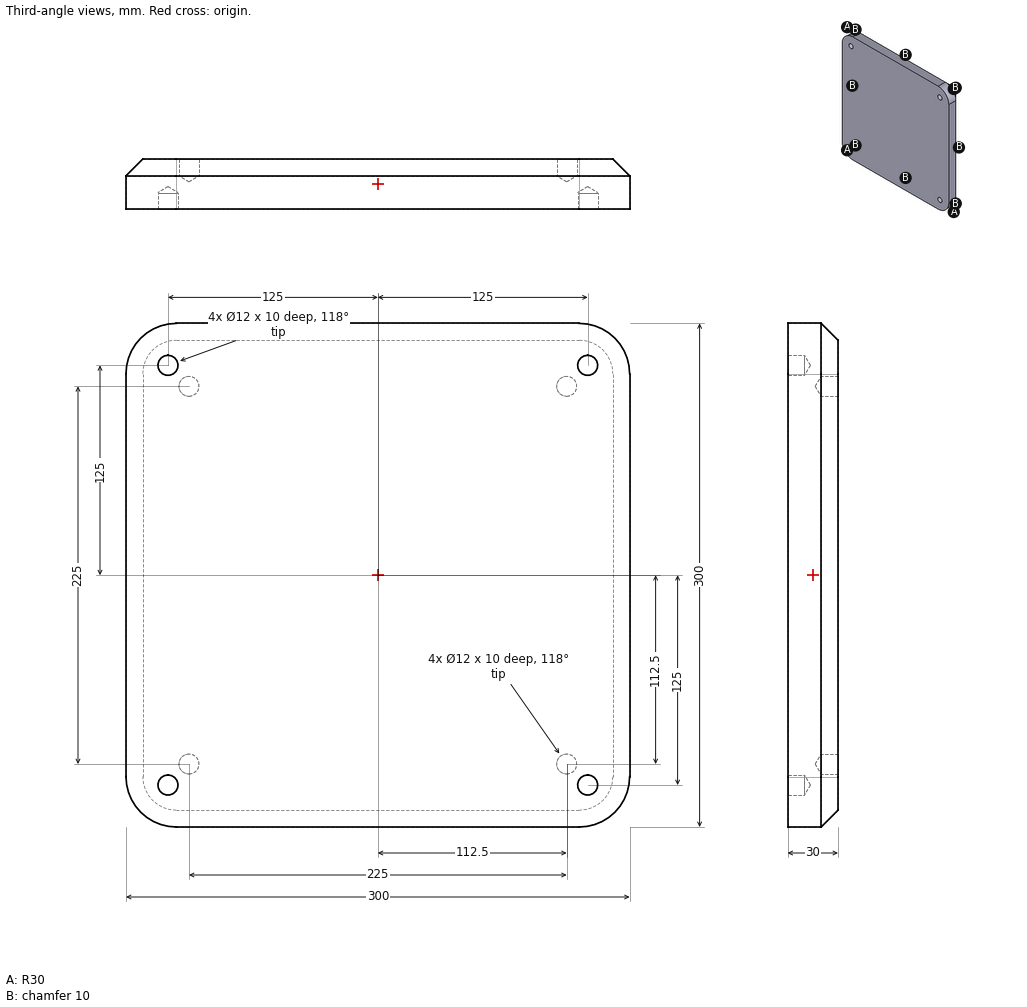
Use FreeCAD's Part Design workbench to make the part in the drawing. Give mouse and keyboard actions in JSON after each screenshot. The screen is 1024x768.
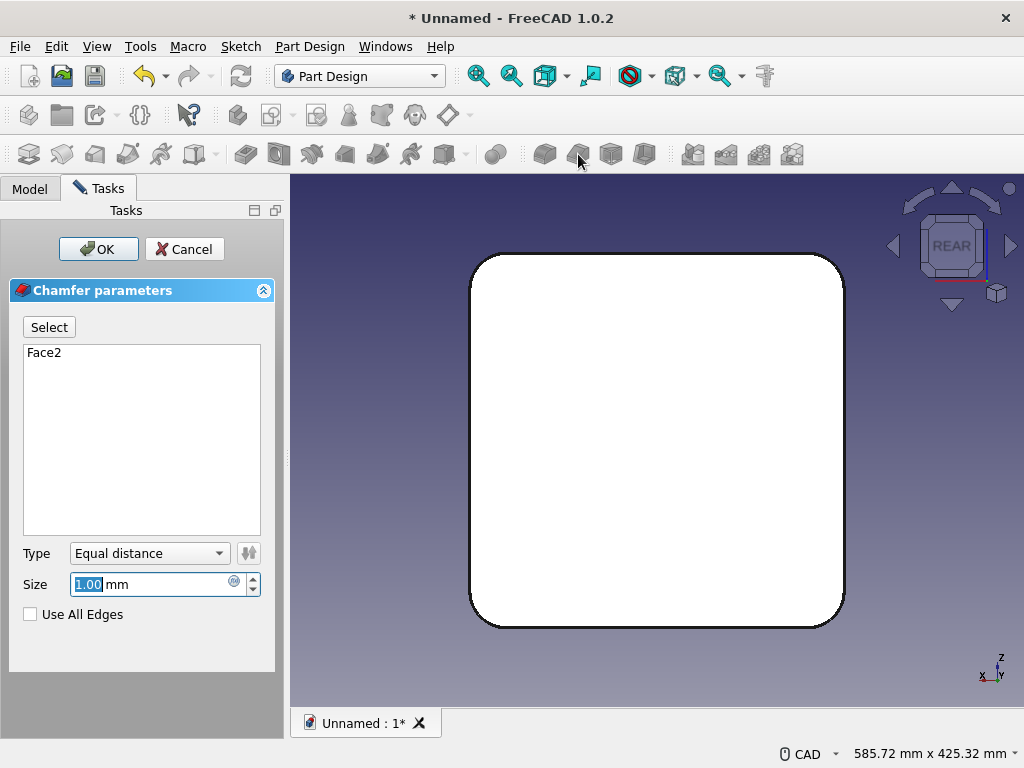
{"action": "type", "text": "10"}
{"action": "key", "text": "Tab"}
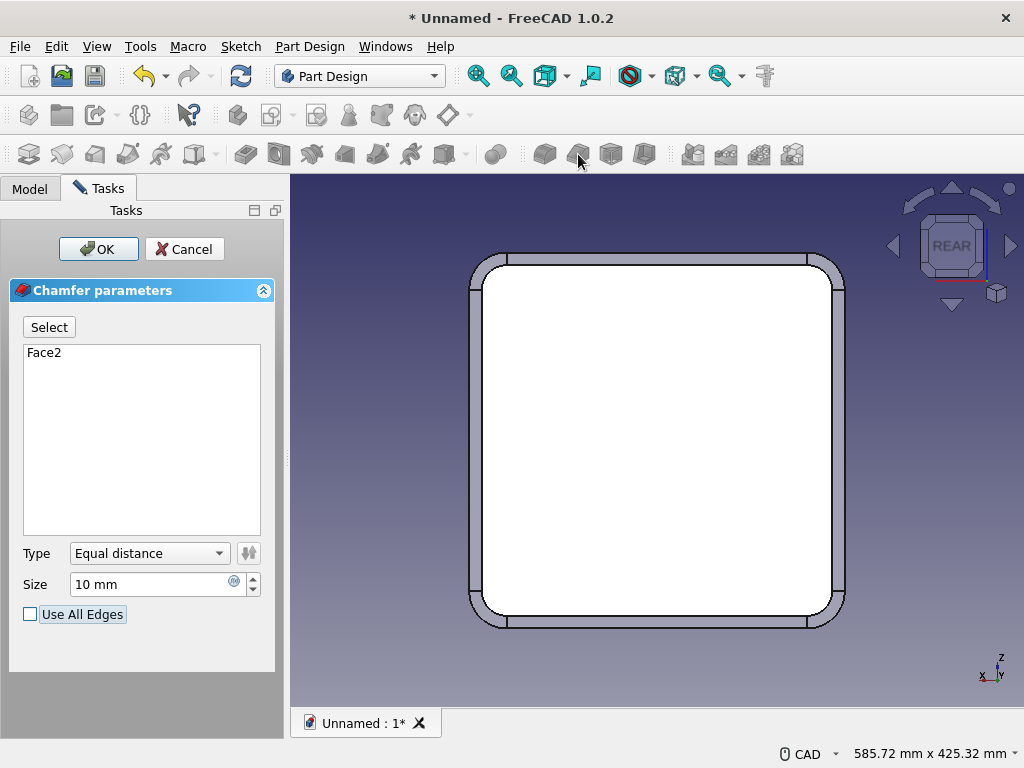
{"action": "left_click", "coordinate": [99, 249]}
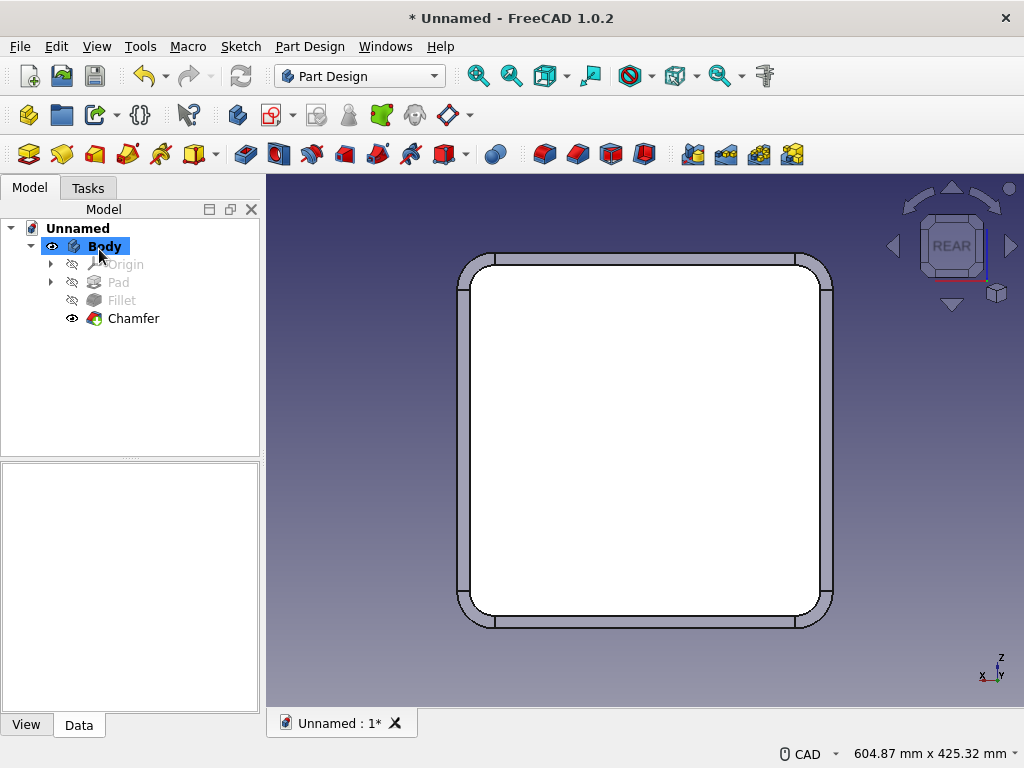
{"action": "left_click", "coordinate": [645, 439]}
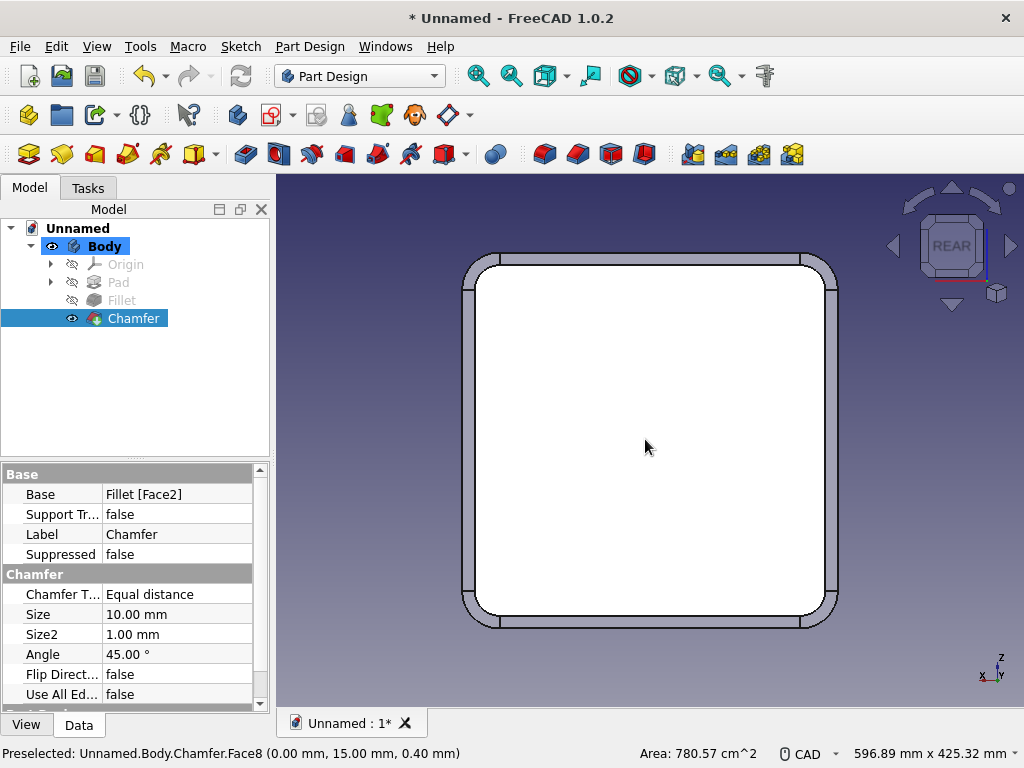
{"action": "left_click", "coordinate": [270, 116]}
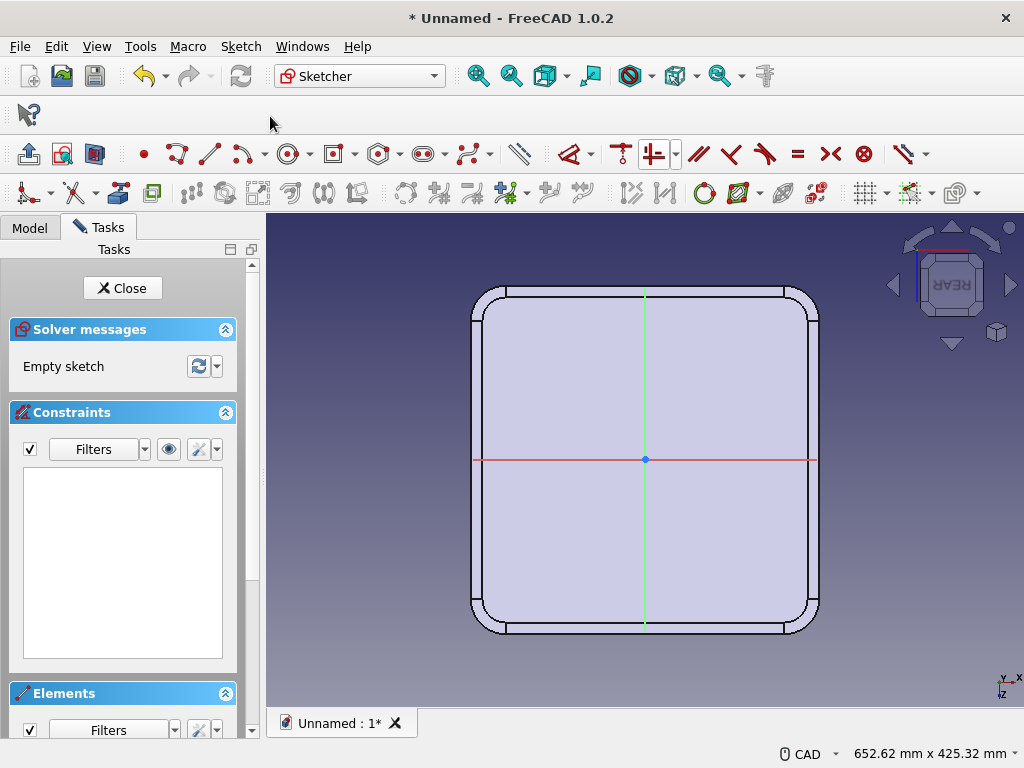
{"action": "left_click", "coordinate": [288, 154]}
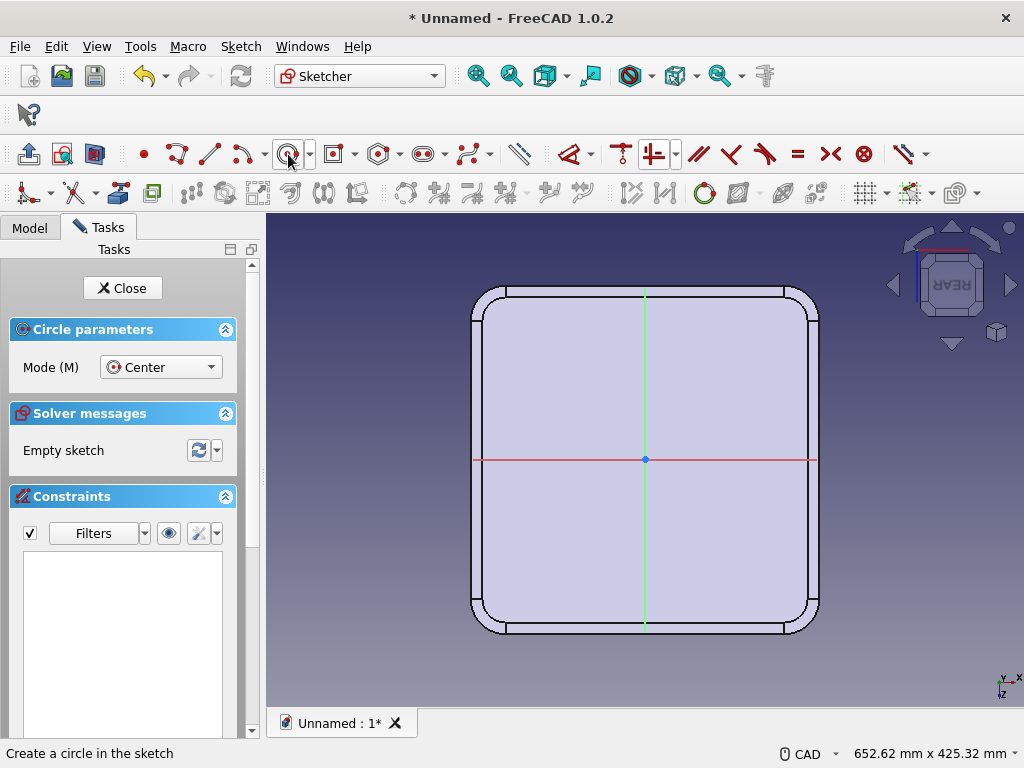
{"action": "scroll", "coordinate": [776, 329], "scroll_direction": "up", "scroll_amount": 6}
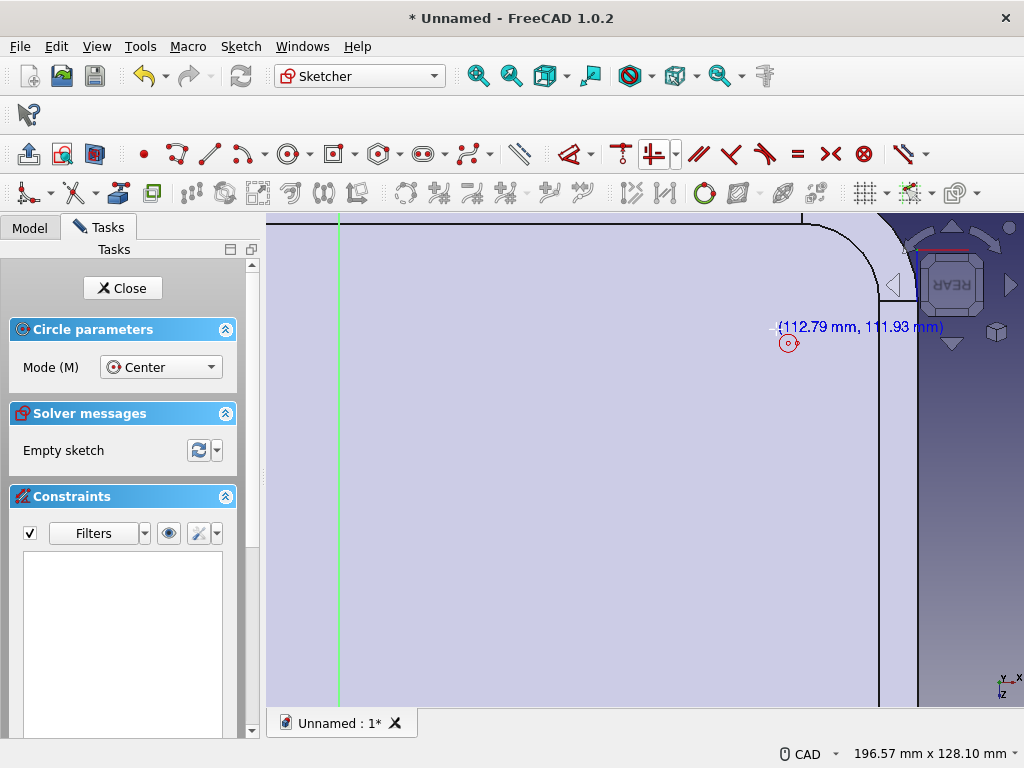
{"action": "left_click", "coordinate": [773, 330]}
{"action": "left_click", "coordinate": [790, 313]}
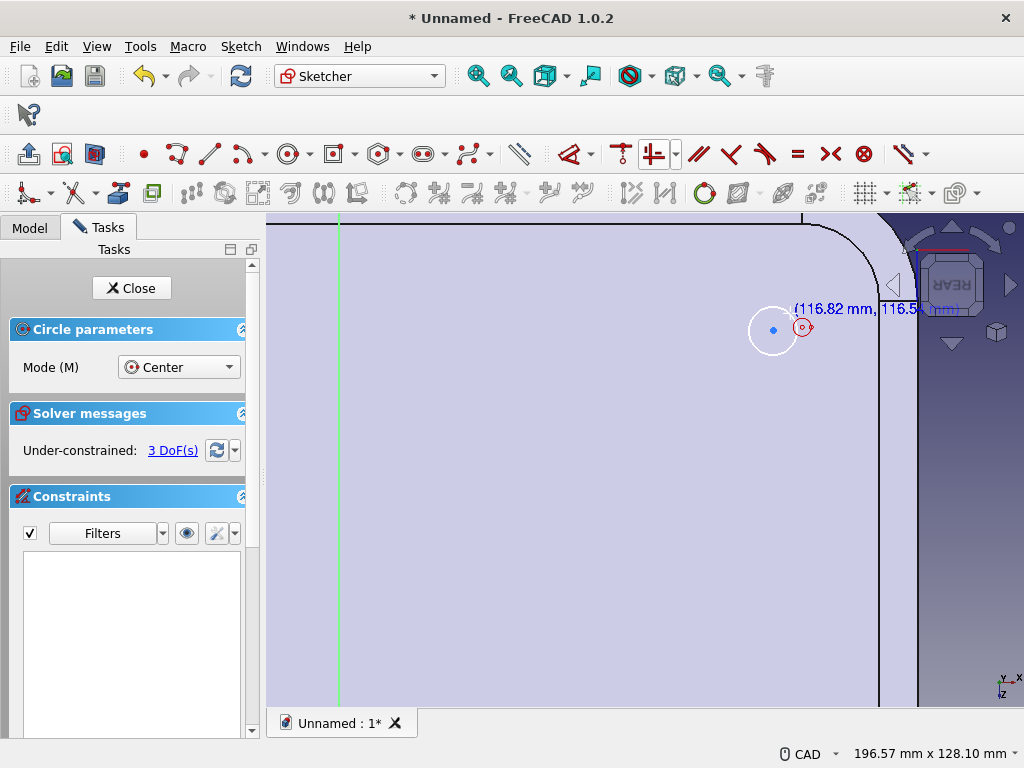
{"action": "scroll", "coordinate": [714, 283], "scroll_direction": "down", "scroll_amount": 5}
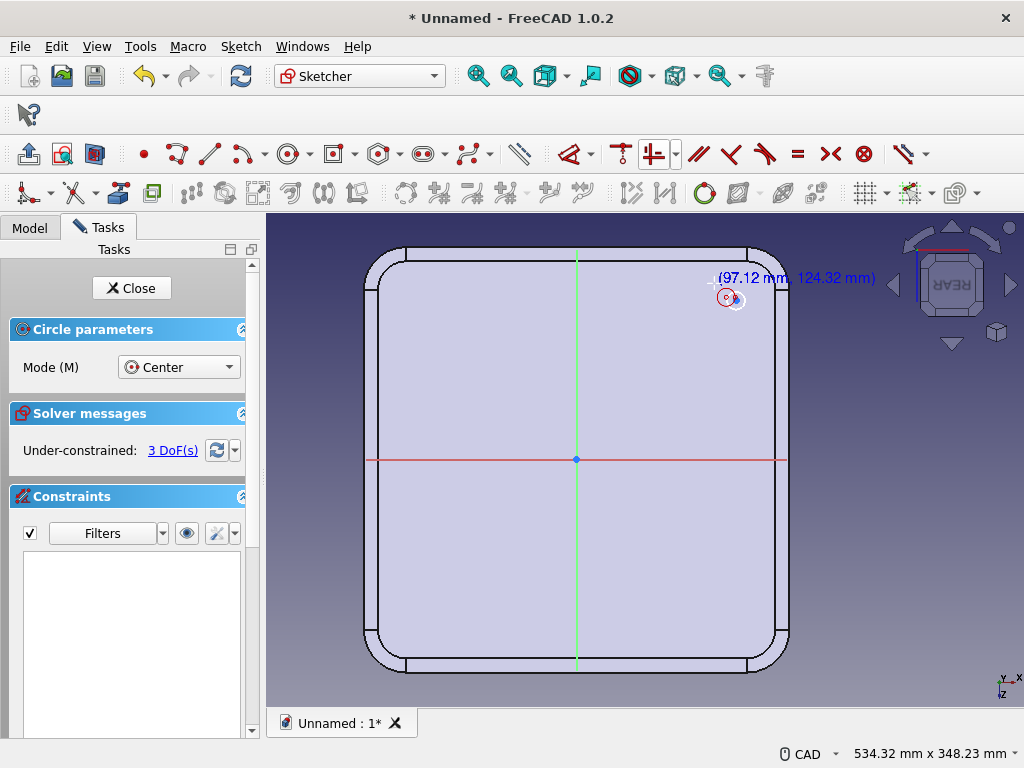
{"action": "scroll", "coordinate": [417, 300], "scroll_direction": "up", "scroll_amount": 5}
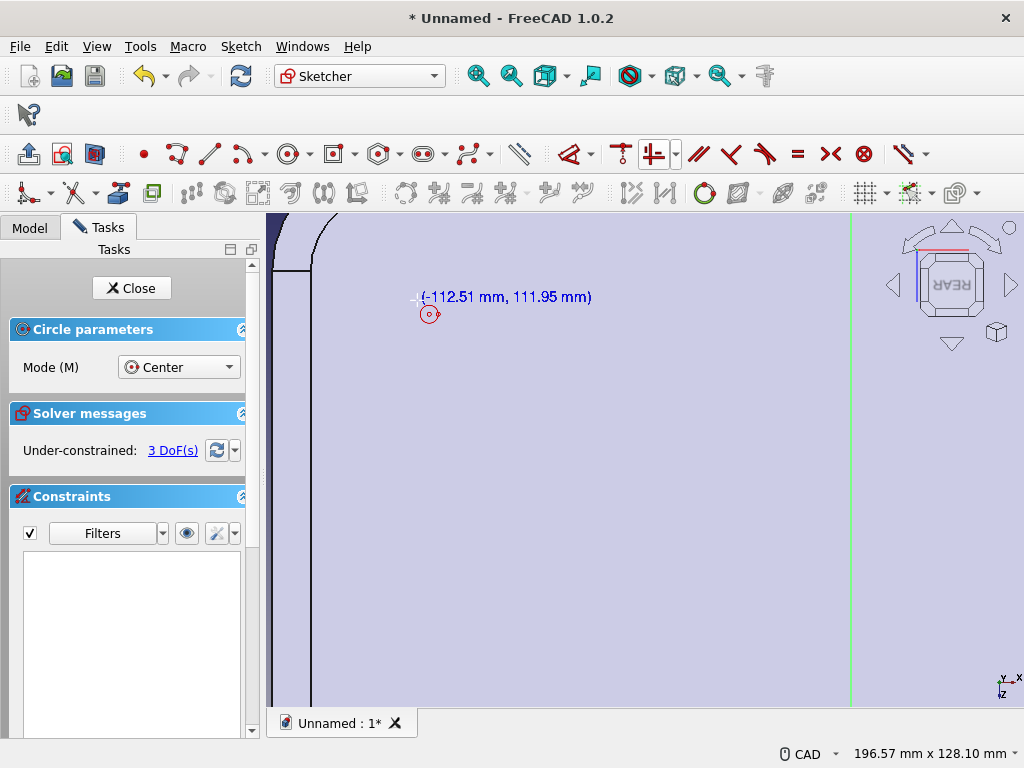
{"action": "left_click", "coordinate": [417, 300]}
{"action": "left_click", "coordinate": [433, 284]}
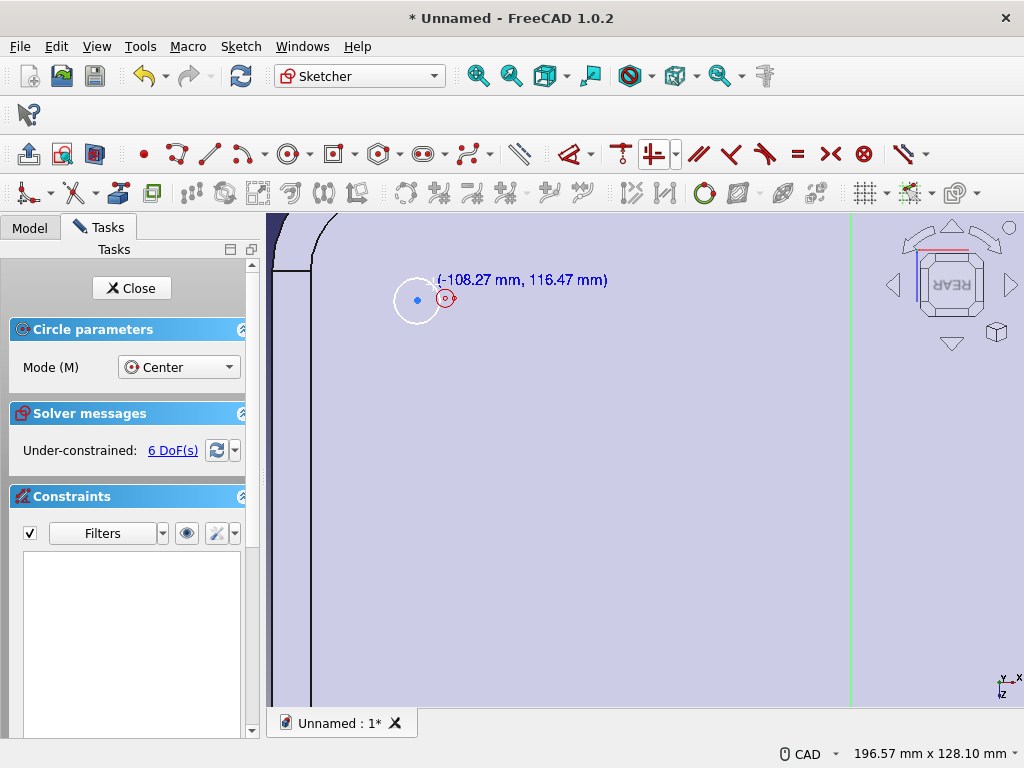
{"action": "scroll", "coordinate": [417, 300], "scroll_direction": "down", "scroll_amount": 5}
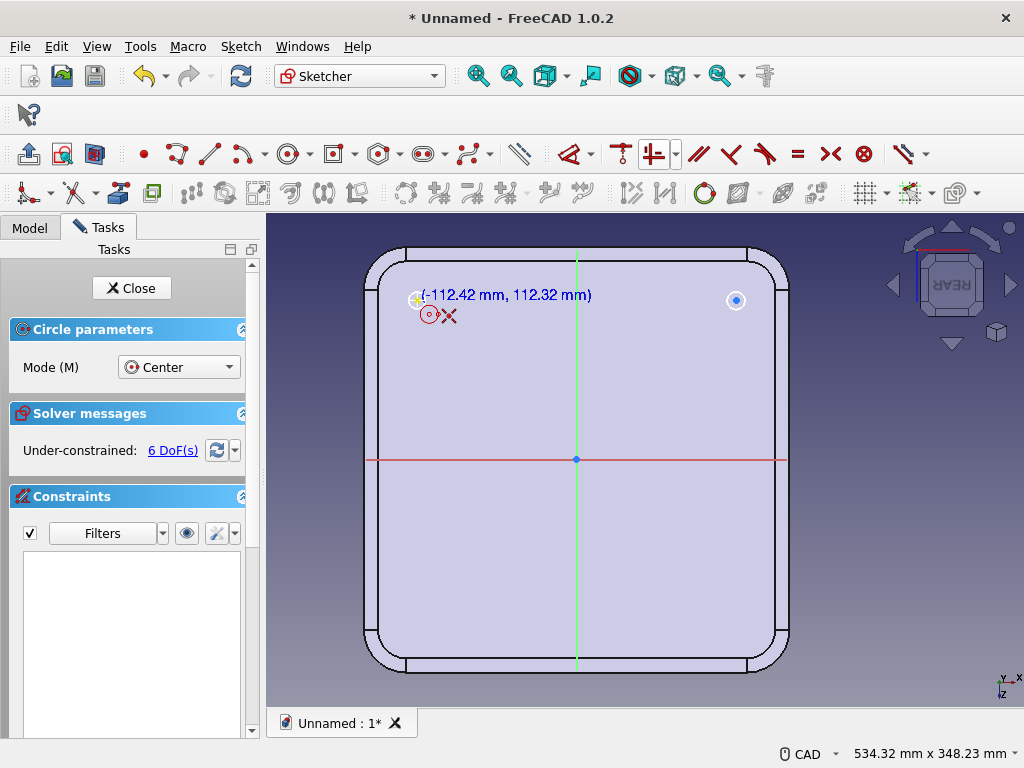
{"action": "scroll", "coordinate": [417, 619], "scroll_direction": "up", "scroll_amount": 5}